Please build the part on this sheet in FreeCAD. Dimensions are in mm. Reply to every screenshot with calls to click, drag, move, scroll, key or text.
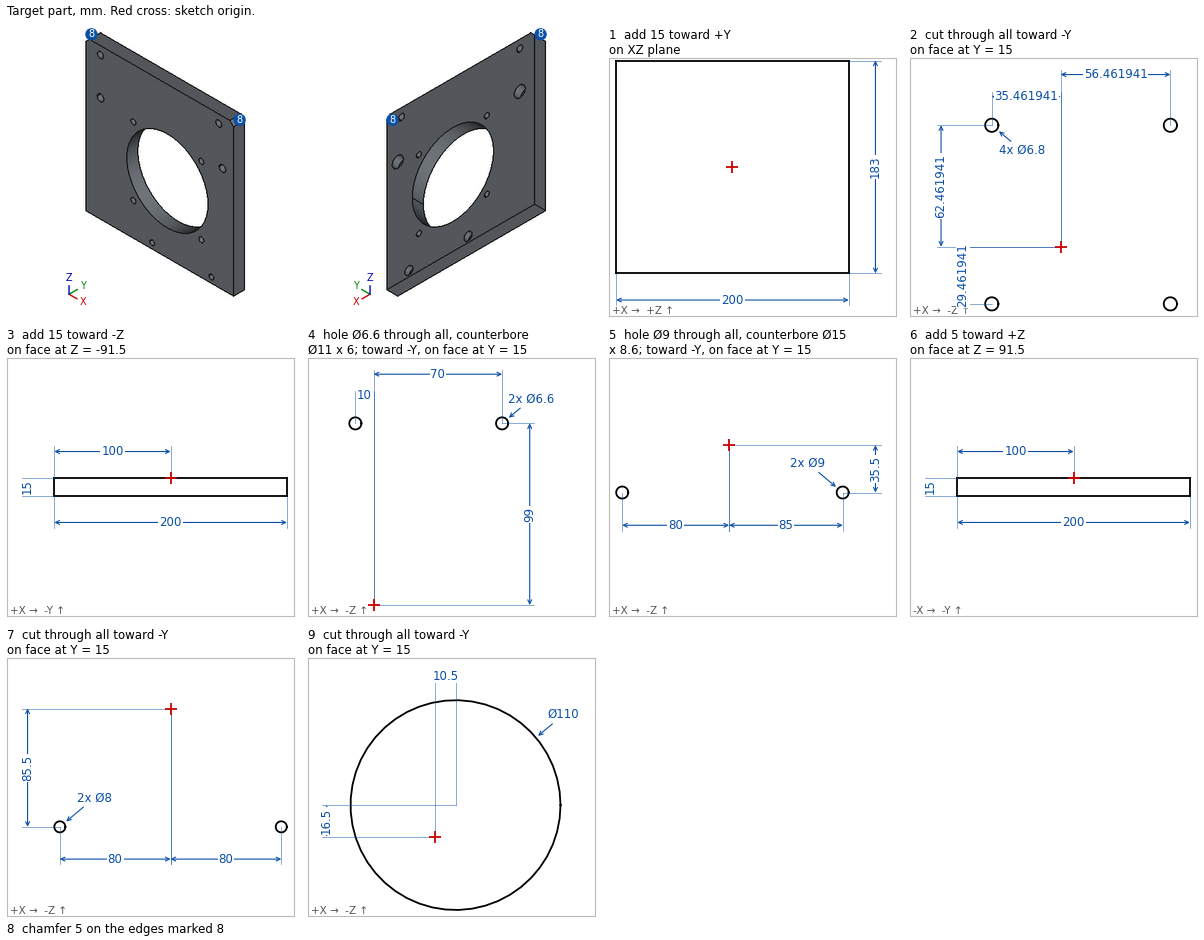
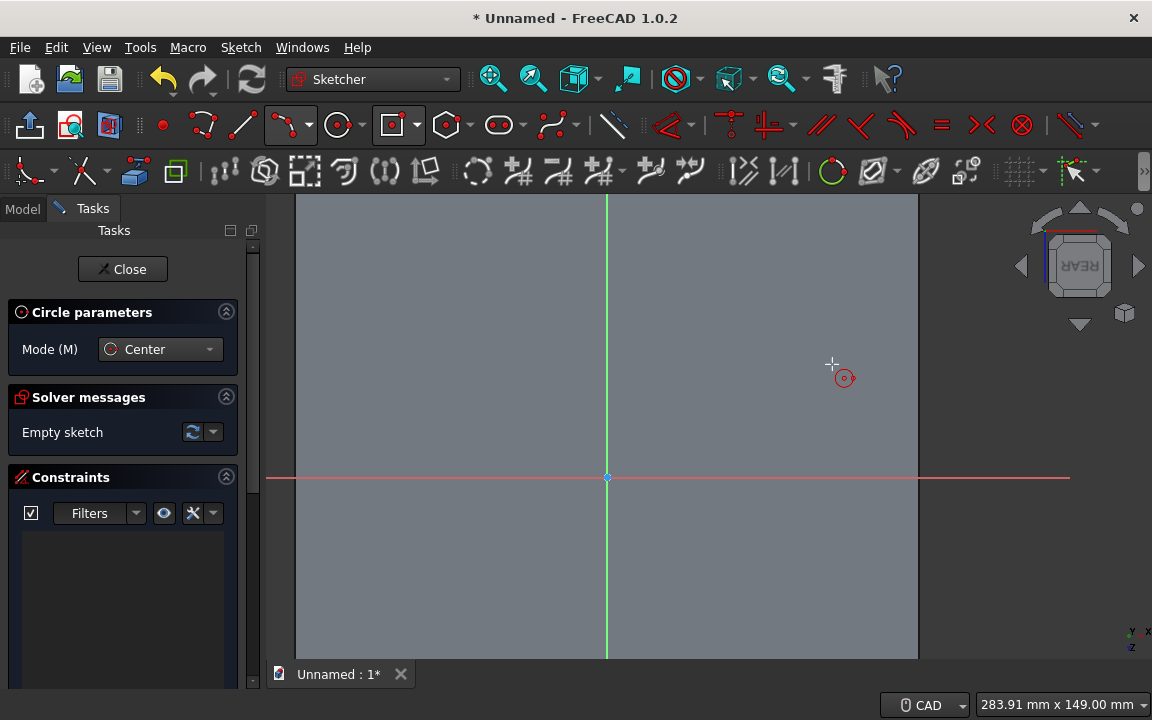
scroll(497, 283, up, 4)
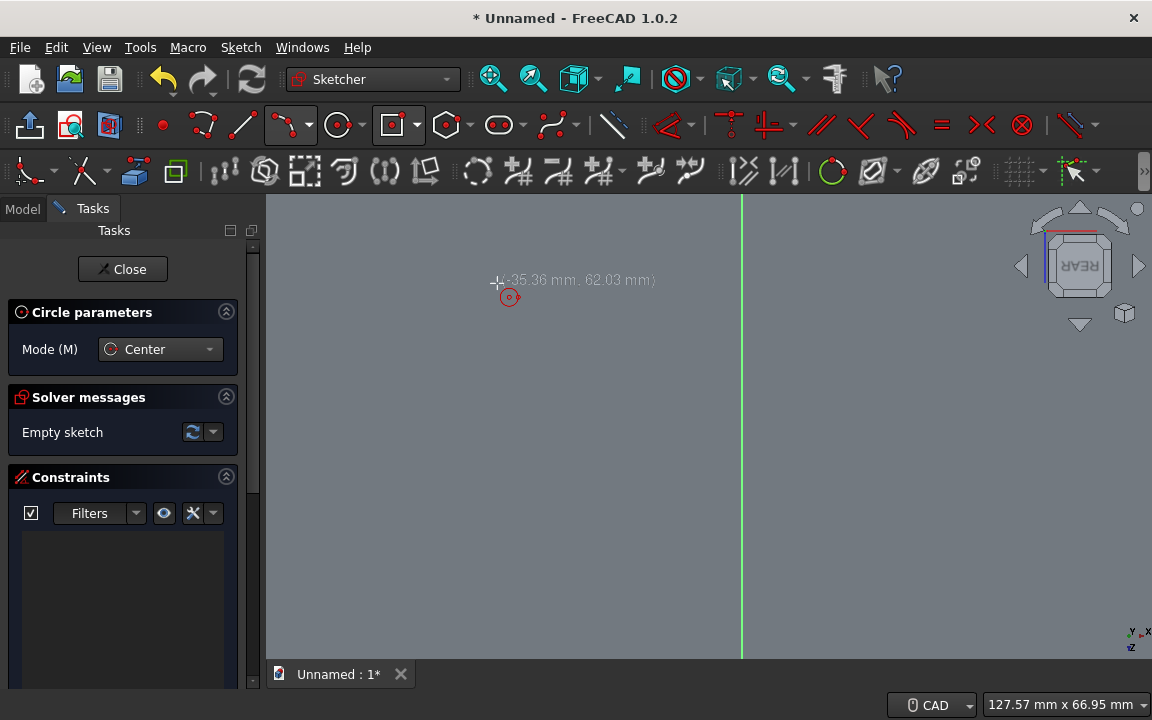
click(496, 282)
click(513, 265)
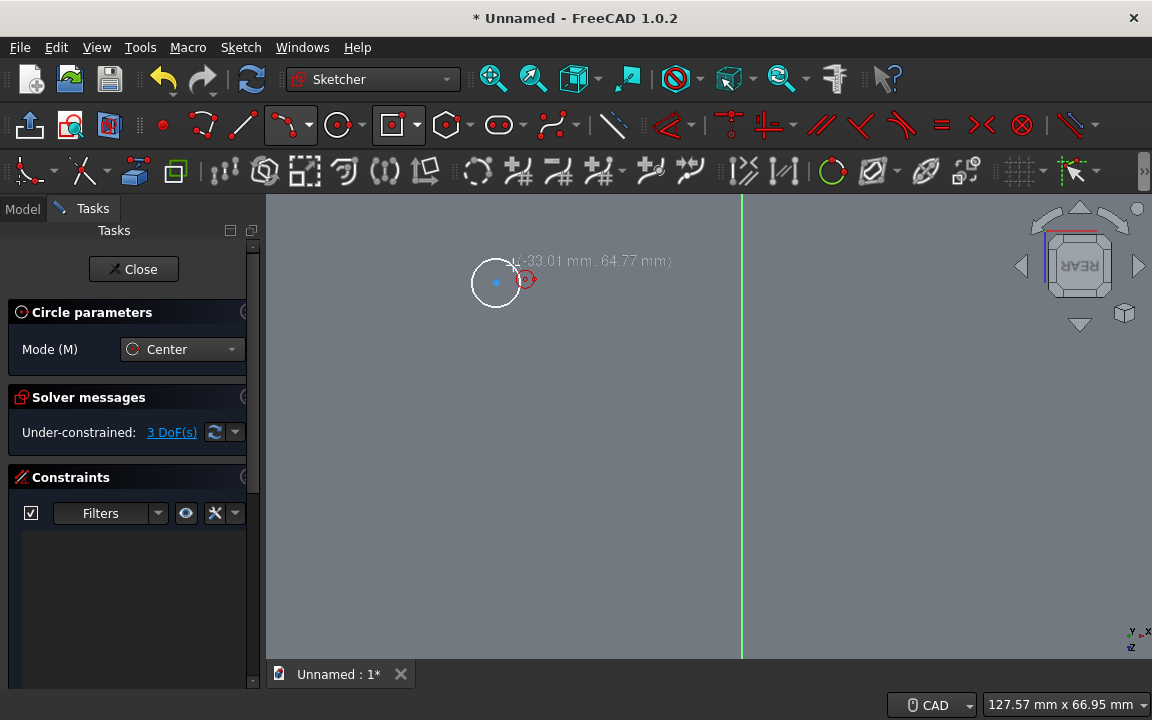
scroll(498, 284, down, 4)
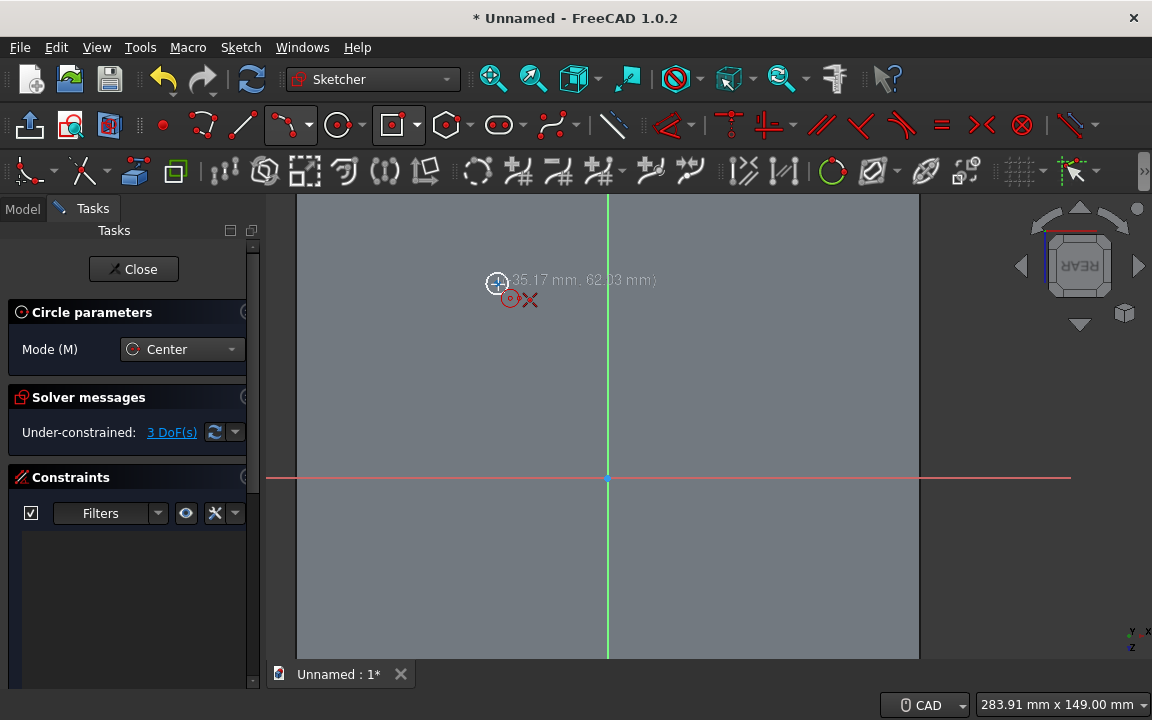
scroll(784, 283, up, 4)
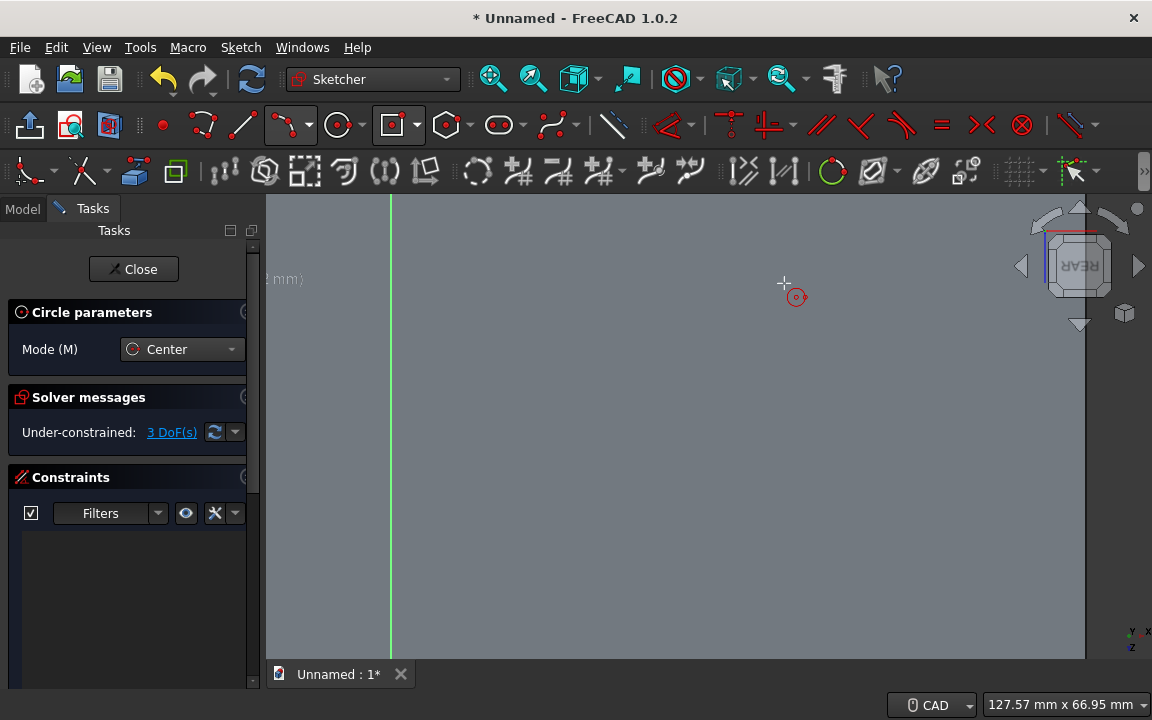
click(784, 283)
click(800, 267)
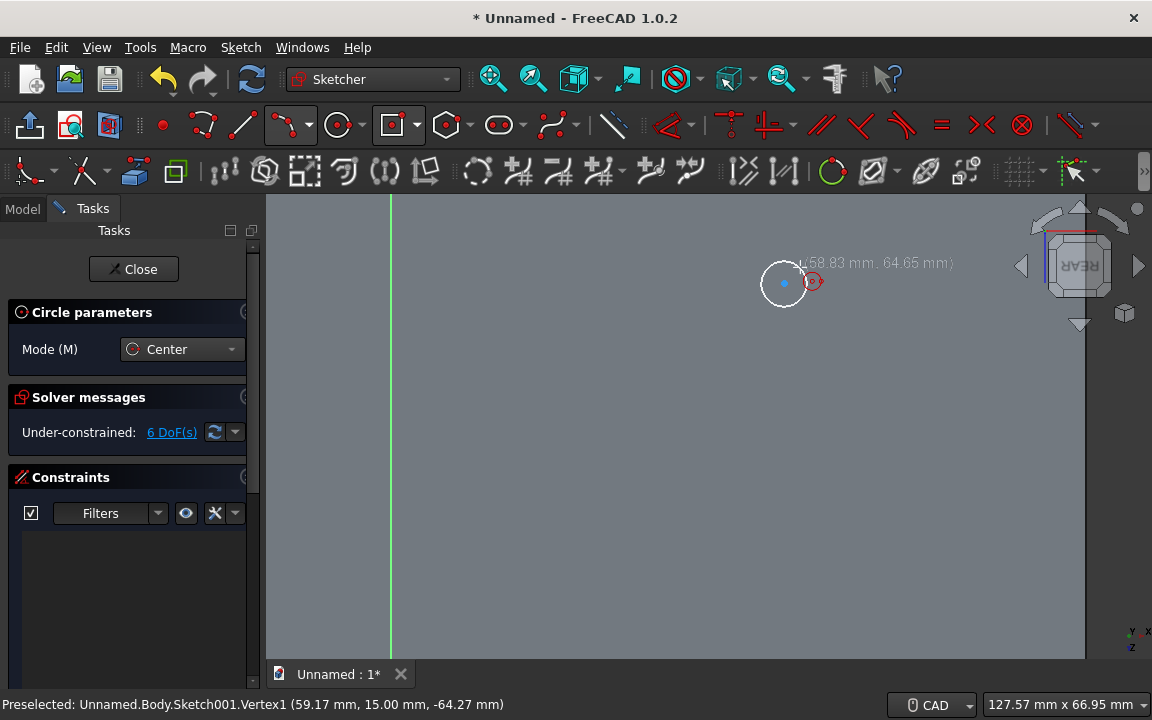
scroll(784, 283, down, 4)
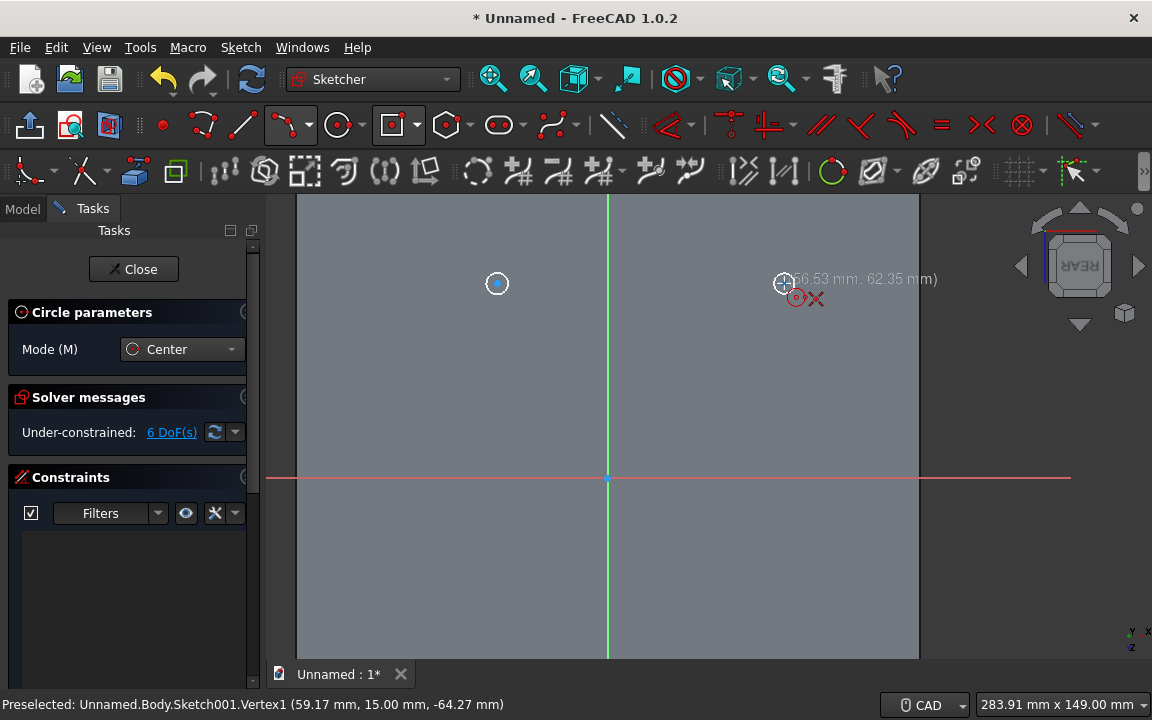
scroll(497, 570, up, 4)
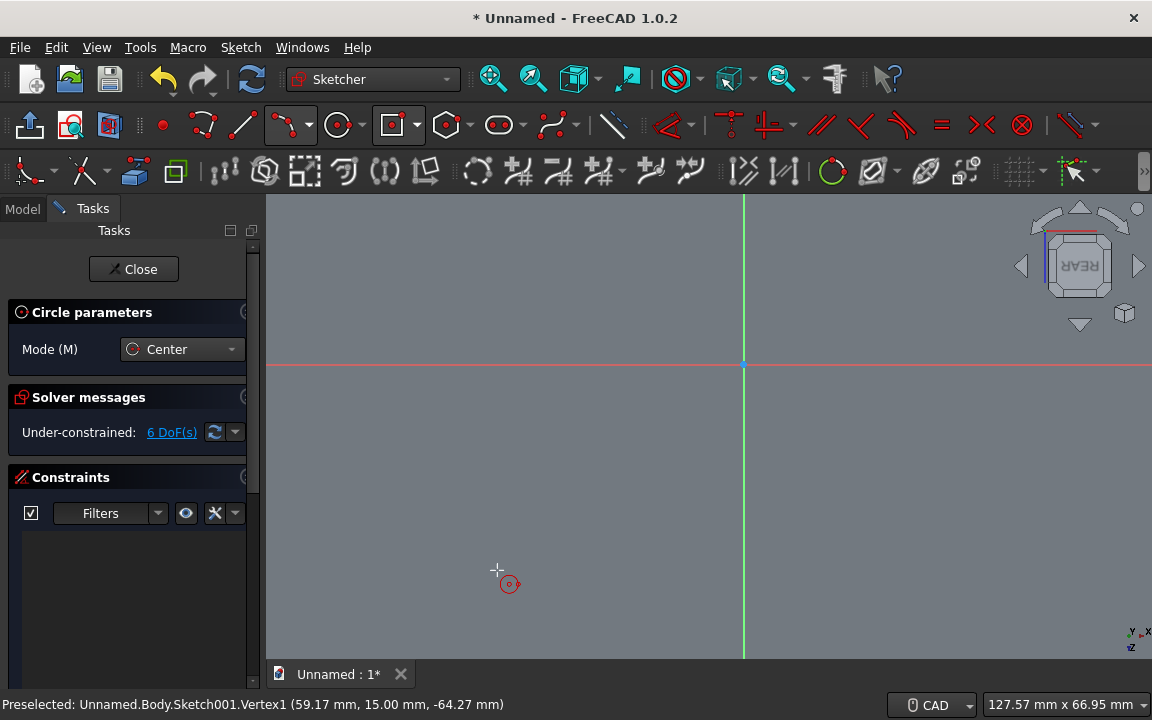
click(497, 569)
click(514, 552)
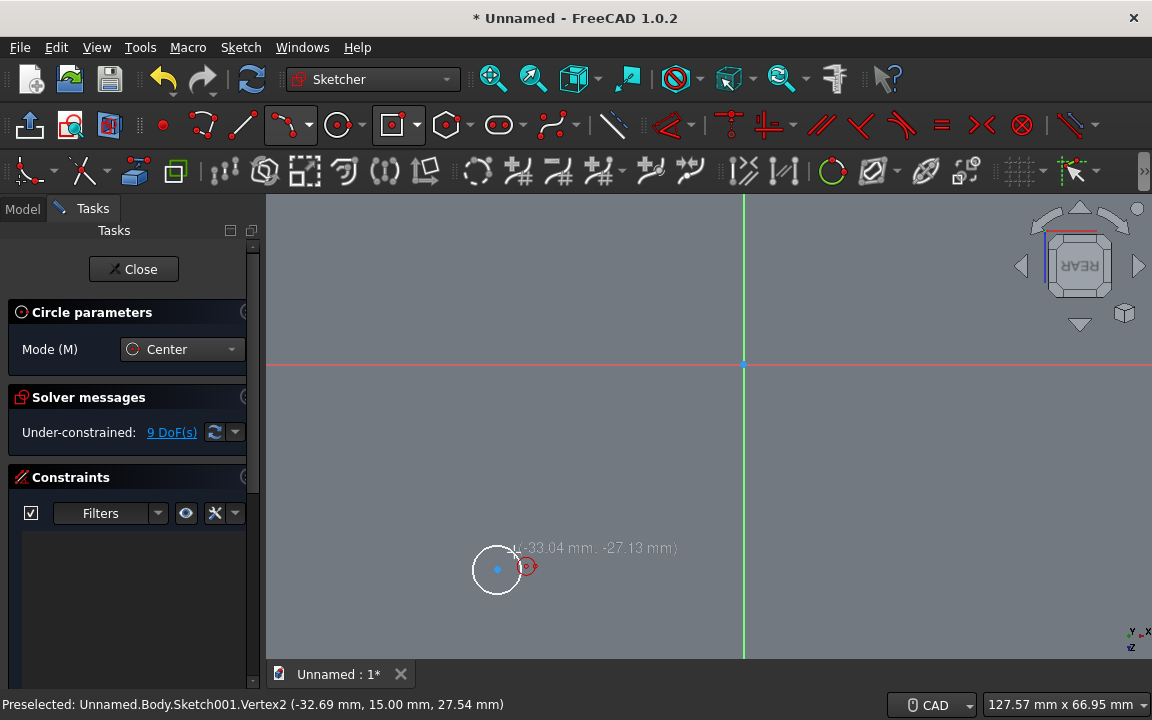
scroll(497, 571, down, 4)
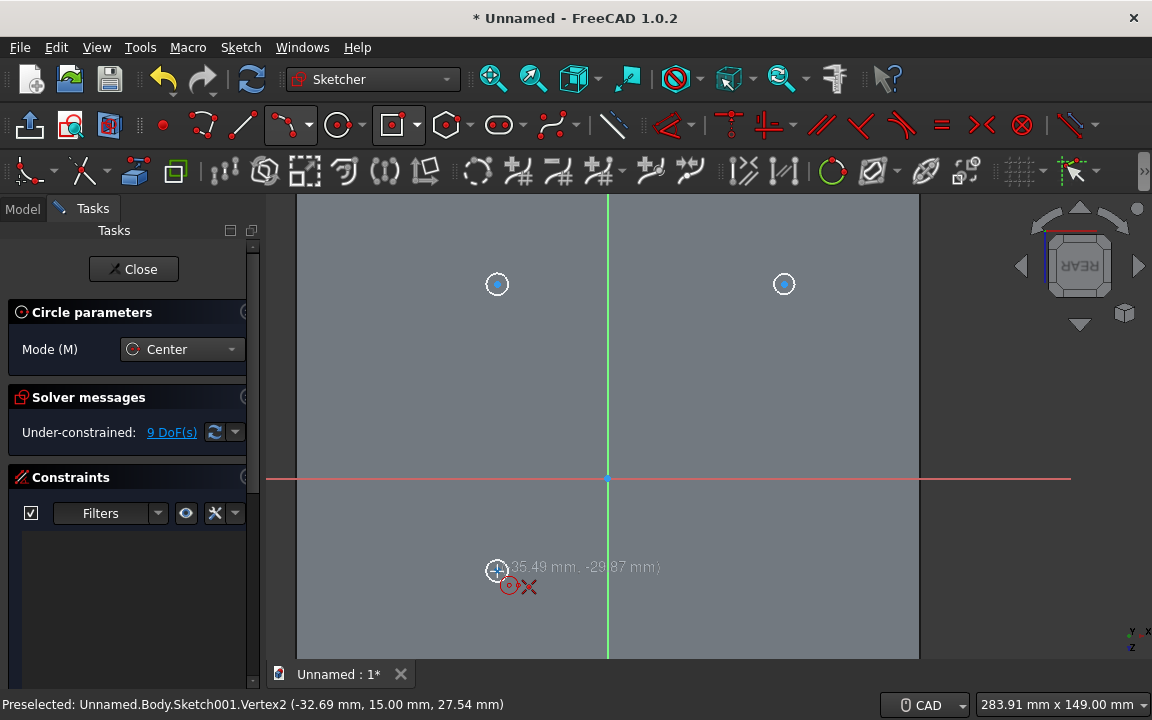
scroll(784, 571, up, 4)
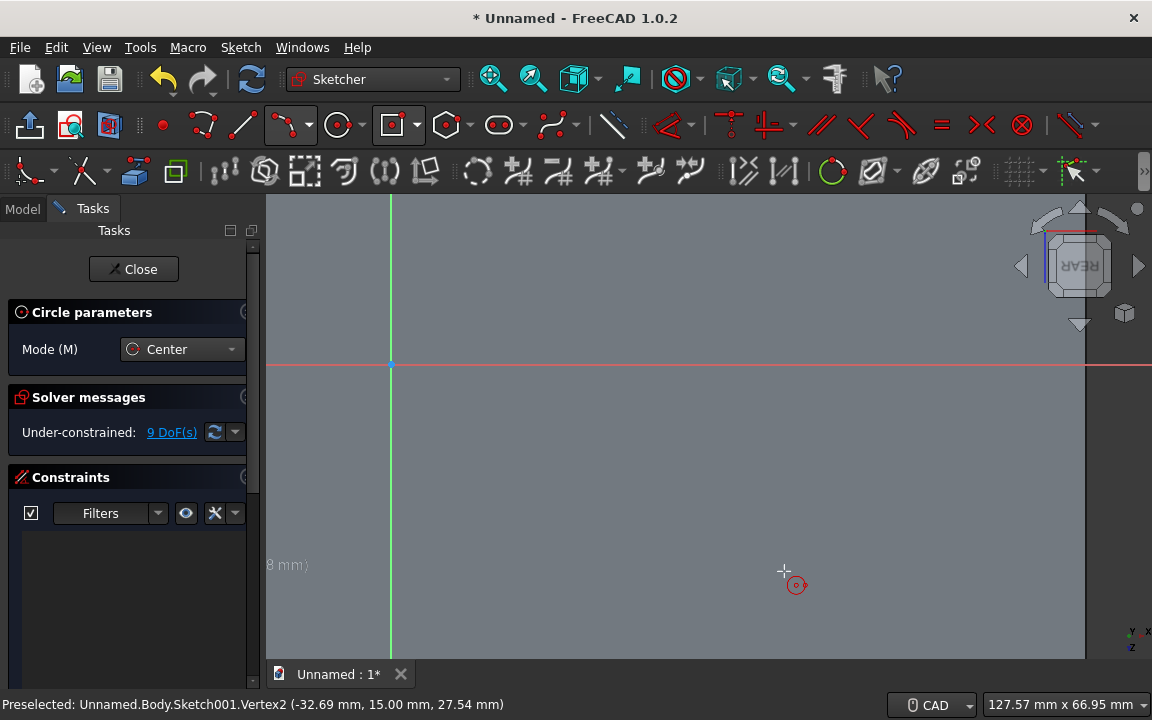
click(784, 569)
click(800, 552)
key(Escape)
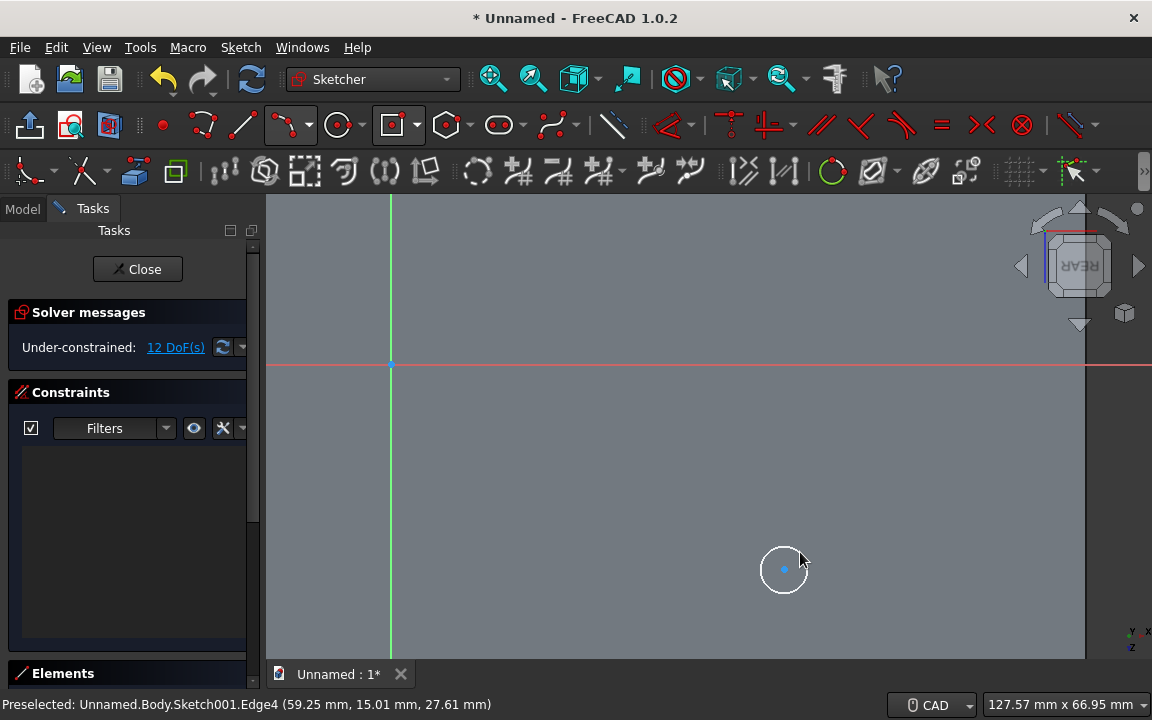
scroll(784, 571, down, 4)